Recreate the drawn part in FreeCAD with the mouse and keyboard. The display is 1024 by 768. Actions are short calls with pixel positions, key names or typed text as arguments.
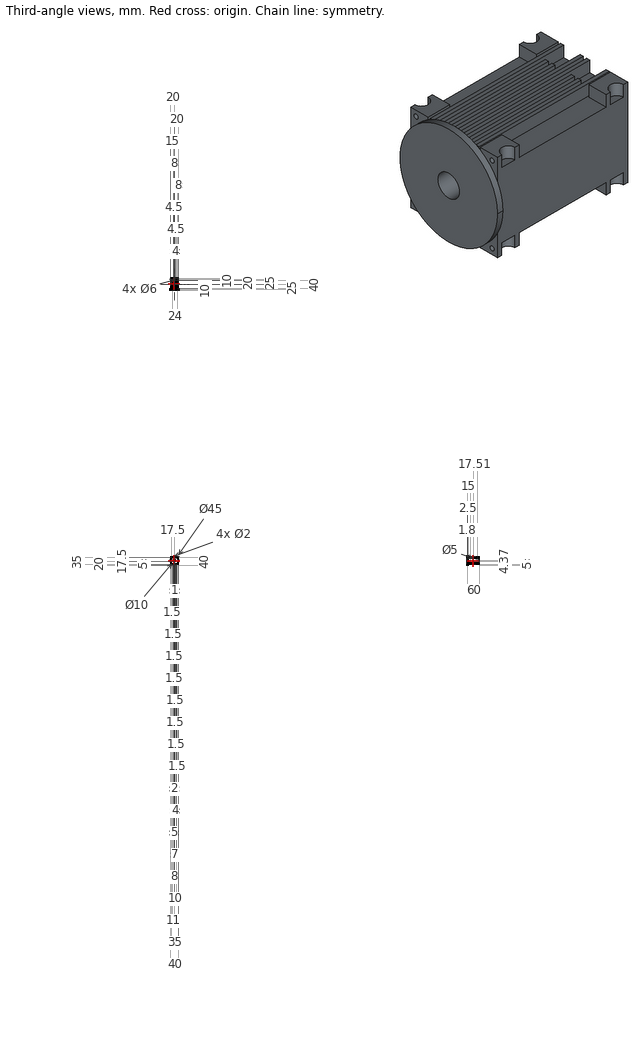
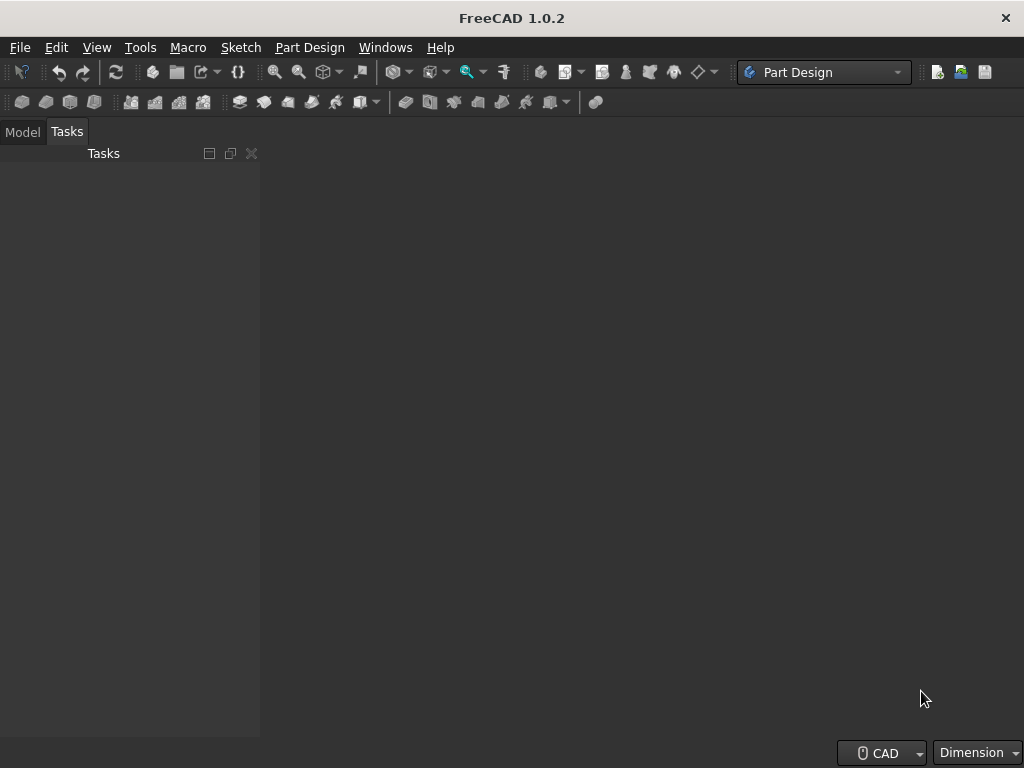
click(938, 72)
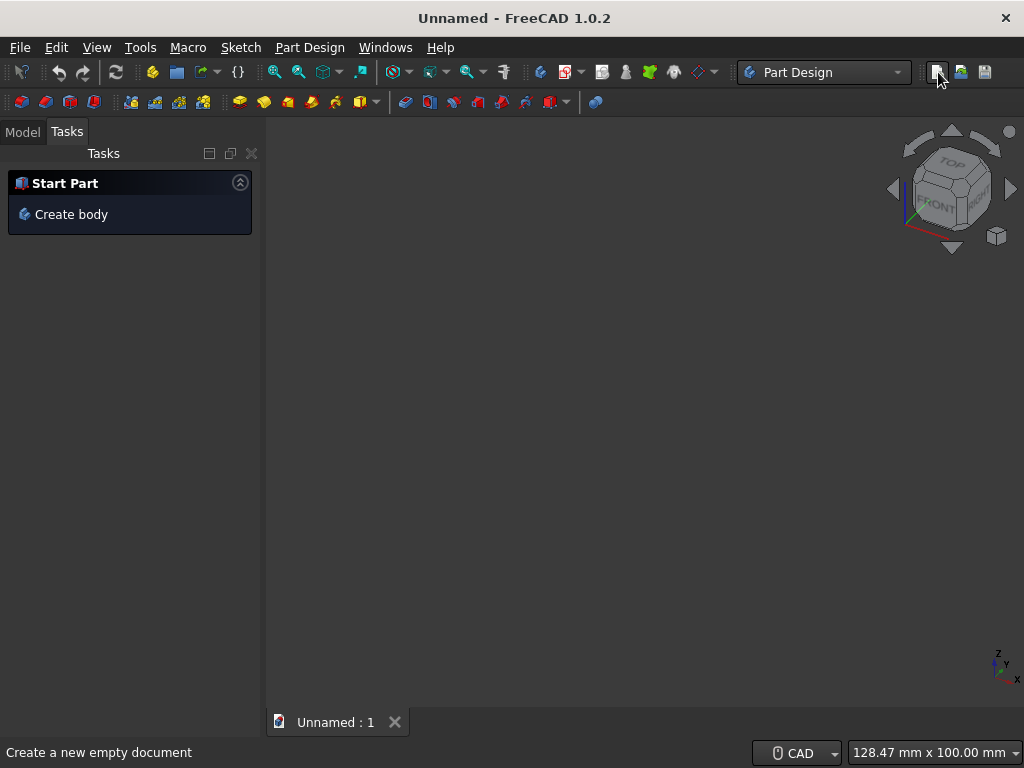
click(566, 72)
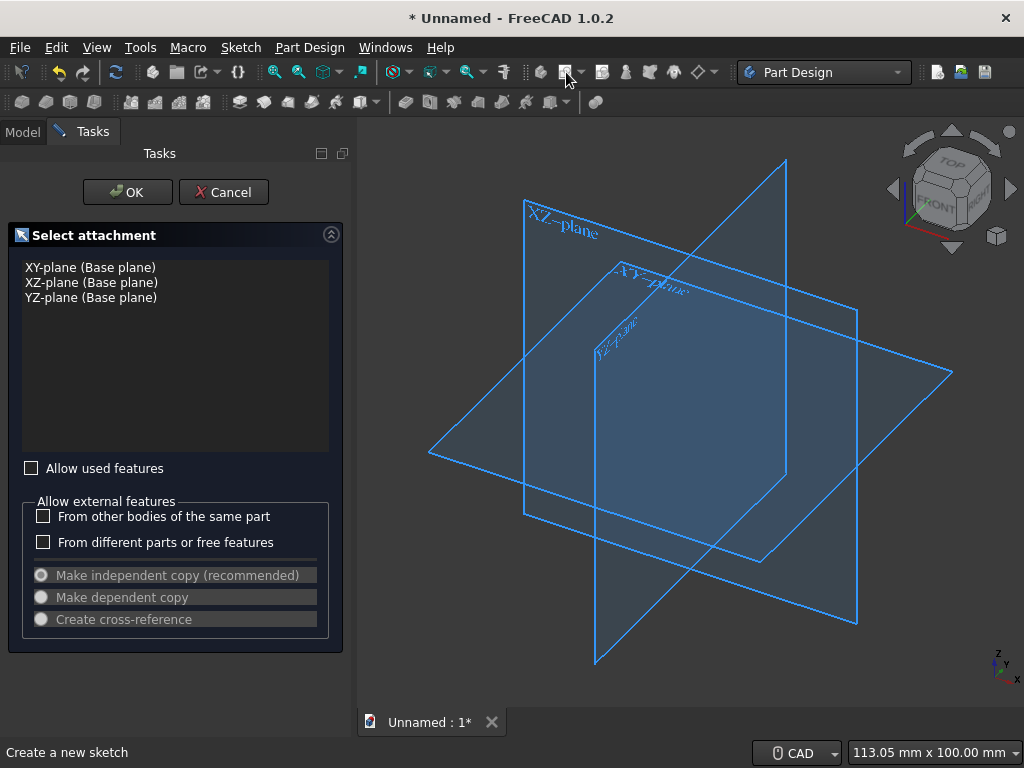
click(82, 282)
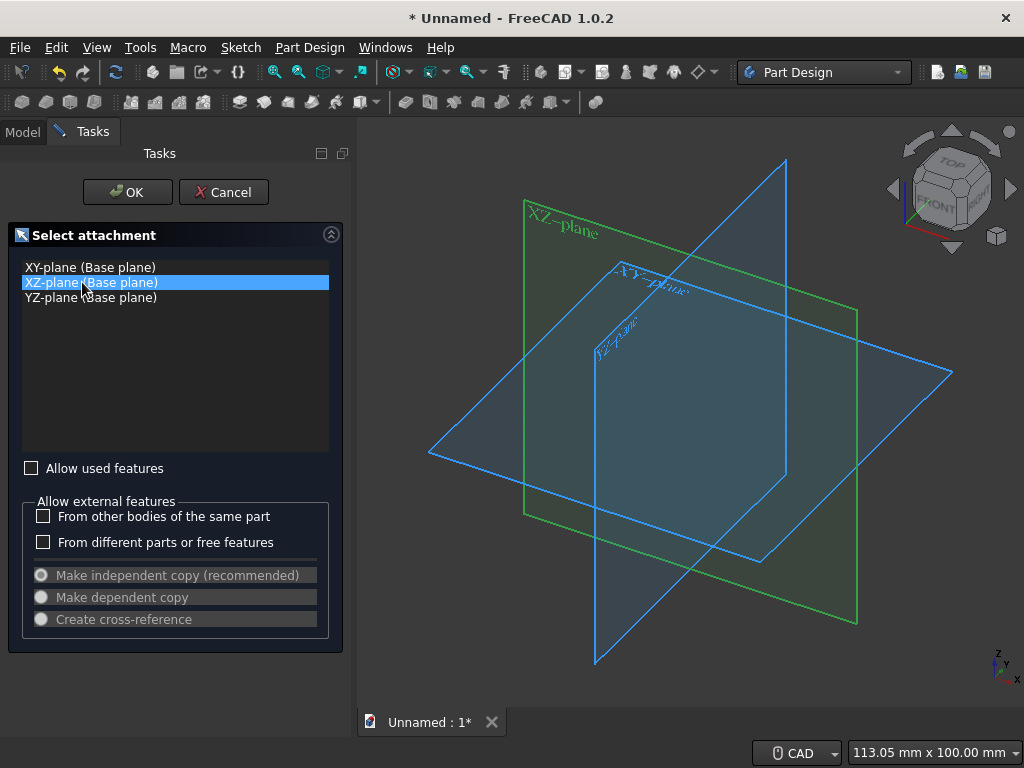
click(128, 192)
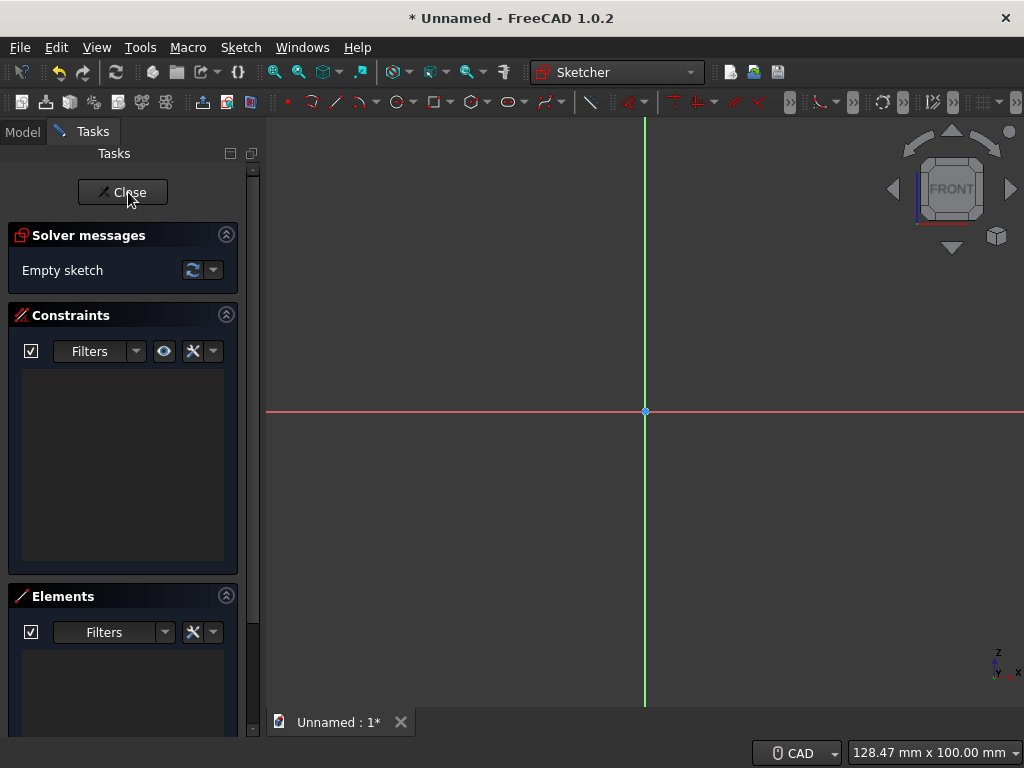
scroll(784, 412, up, 2)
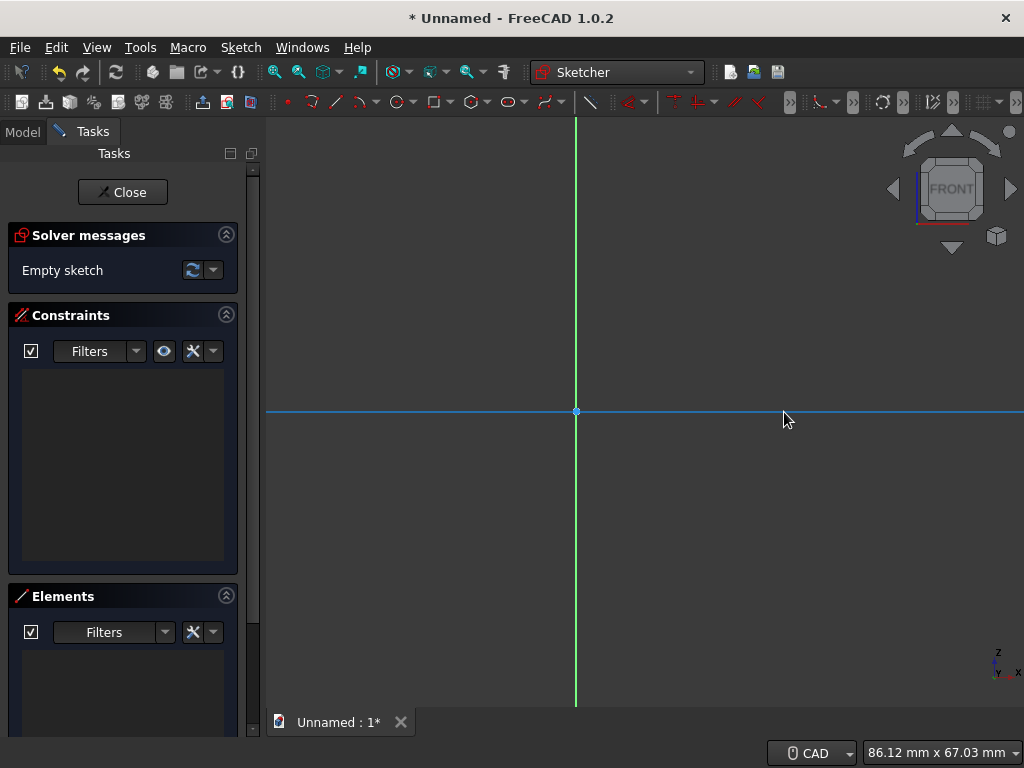
click(452, 102)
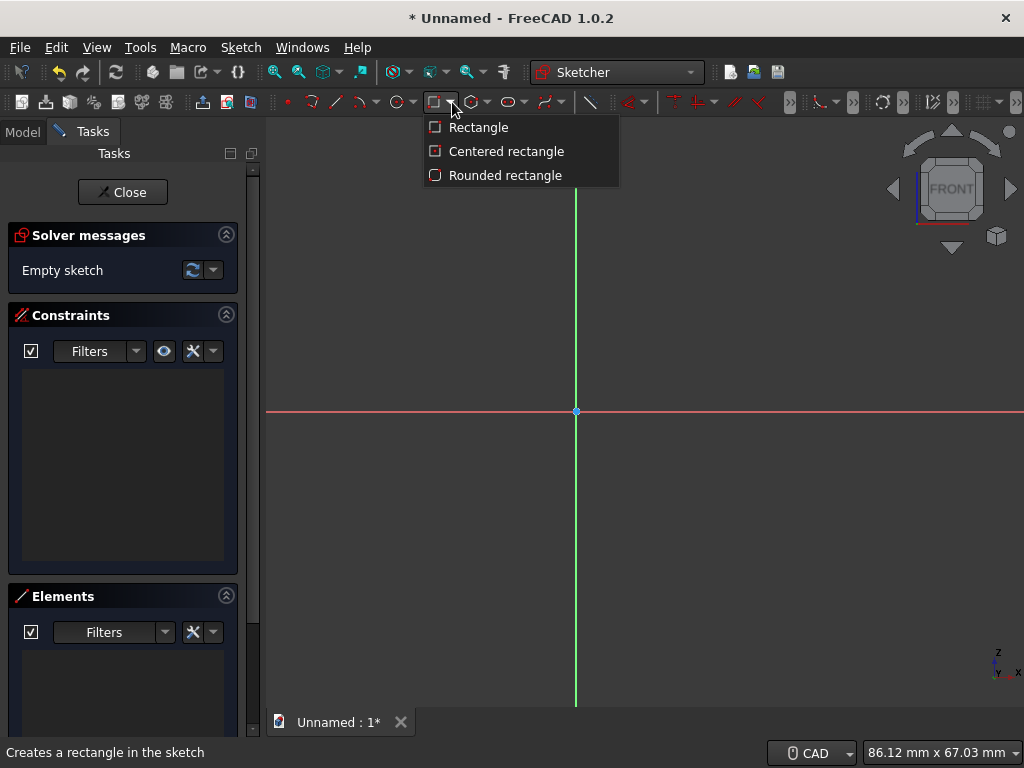
click(522, 151)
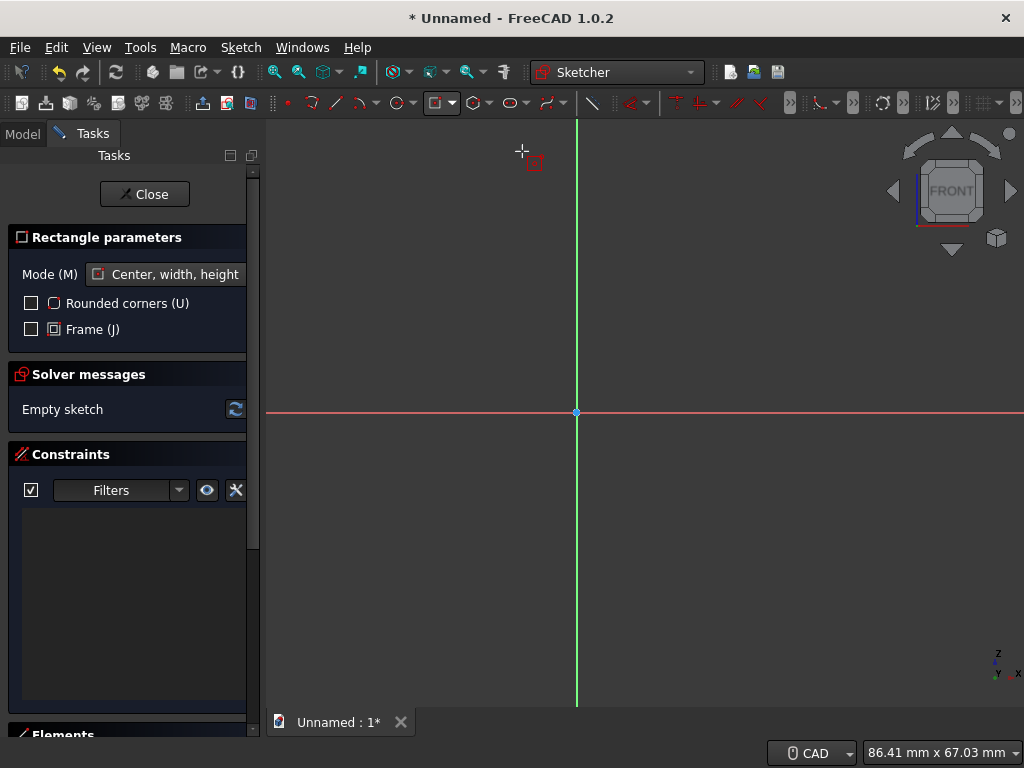
click(577, 413)
click(752, 237)
key(Escape)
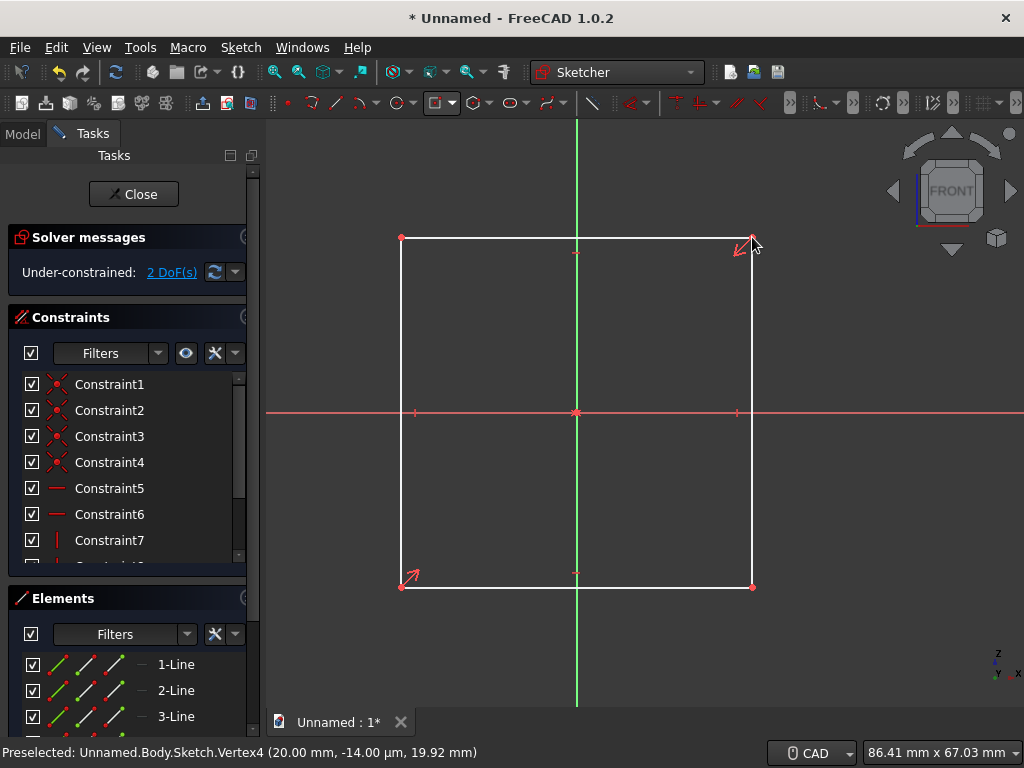
click(630, 104)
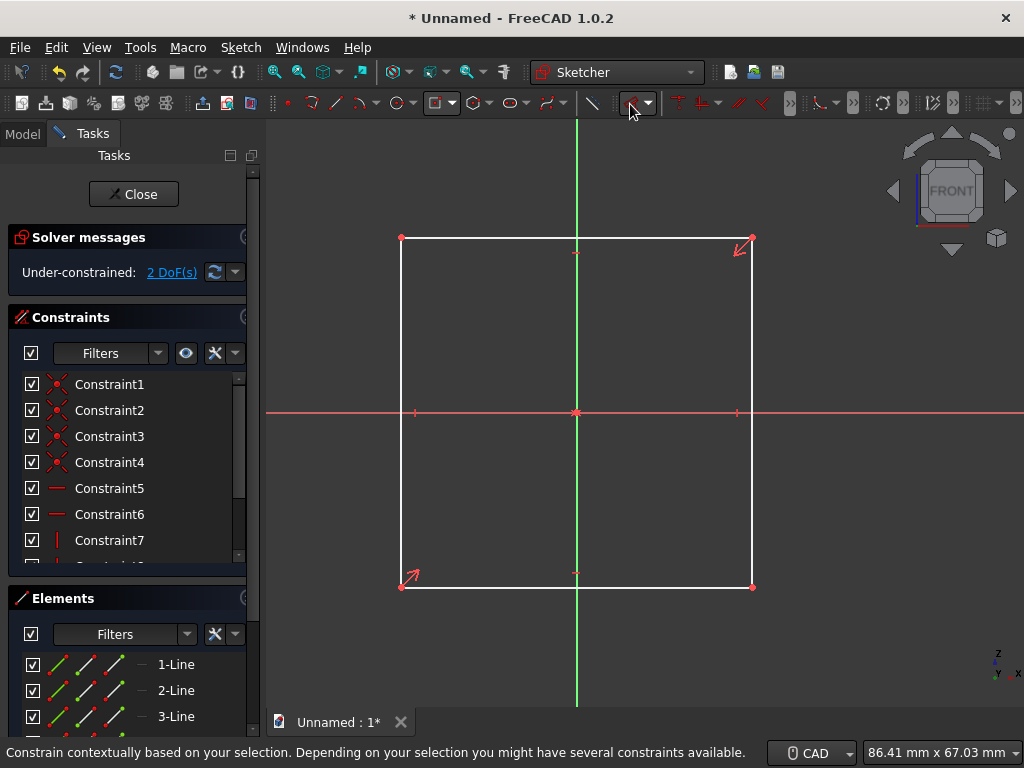
click(506, 588)
click(496, 622)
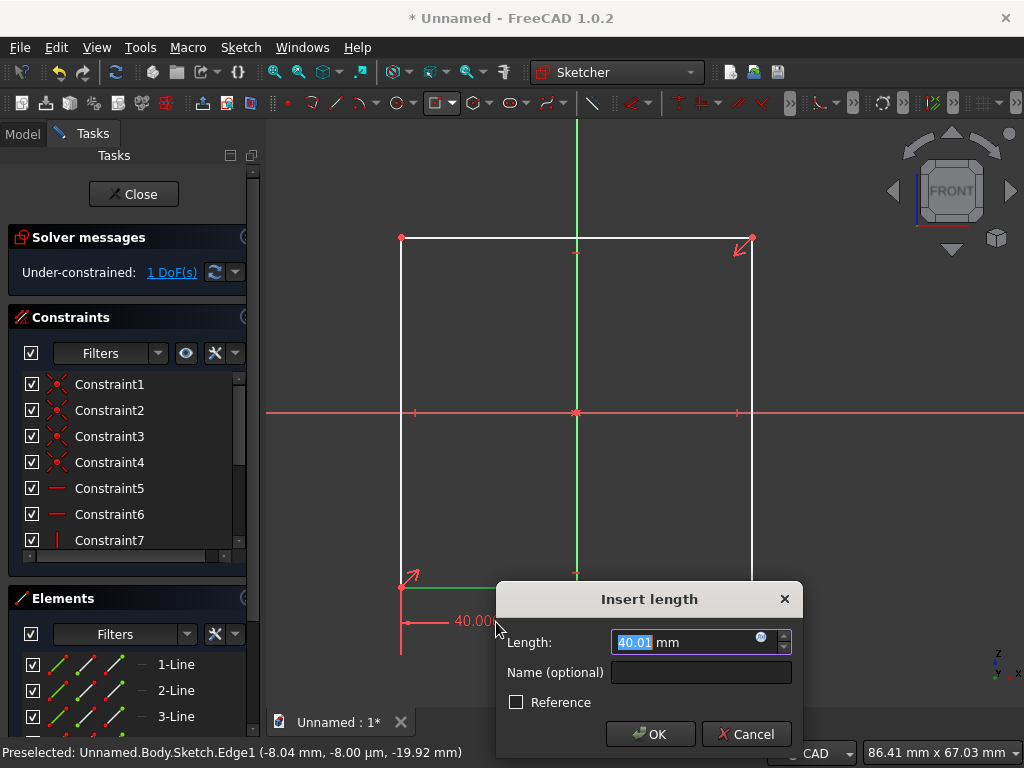
text(40)
key(Return)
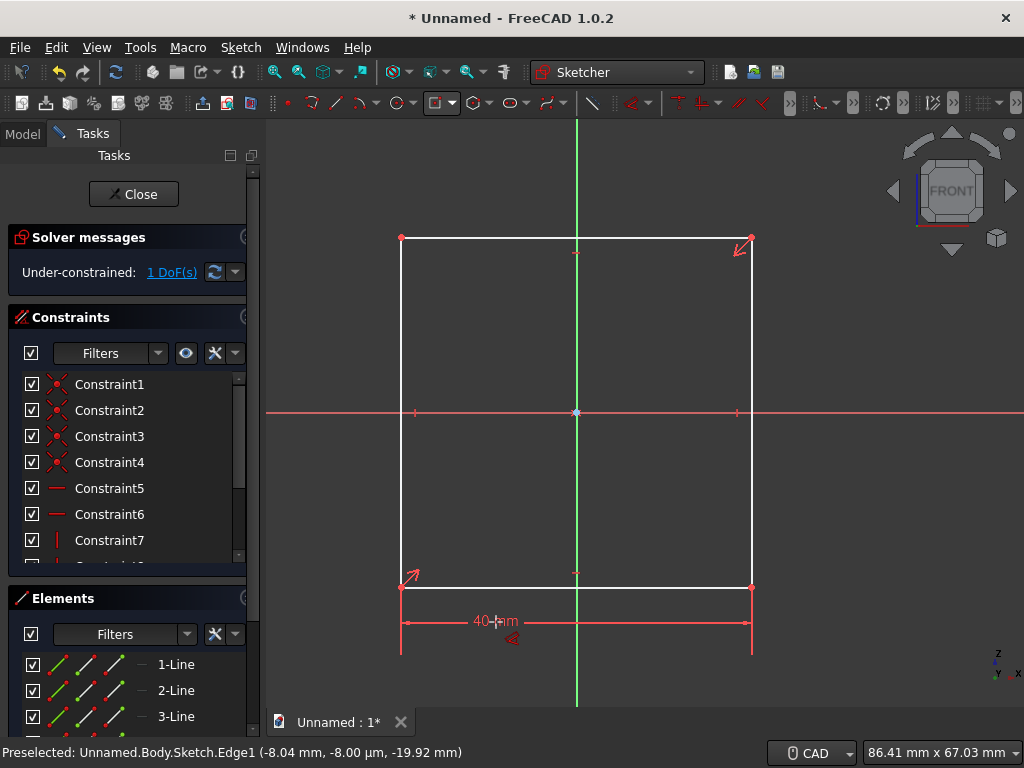
click(752, 483)
click(786, 332)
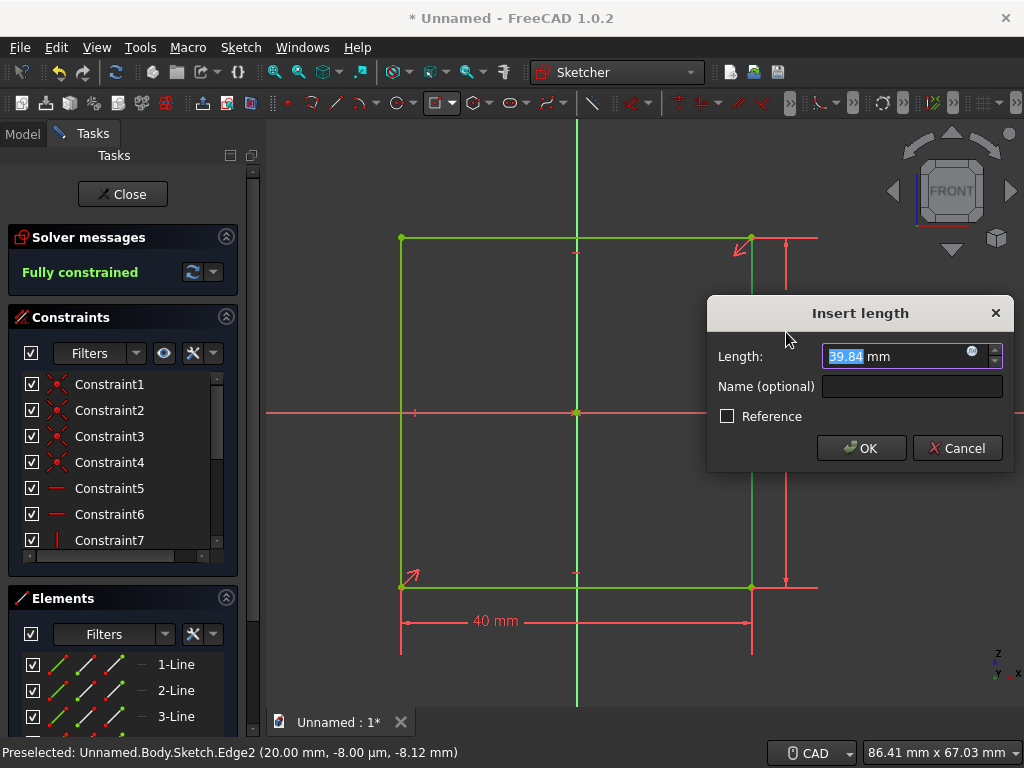
text(40)
key(Return)
key(Escape)